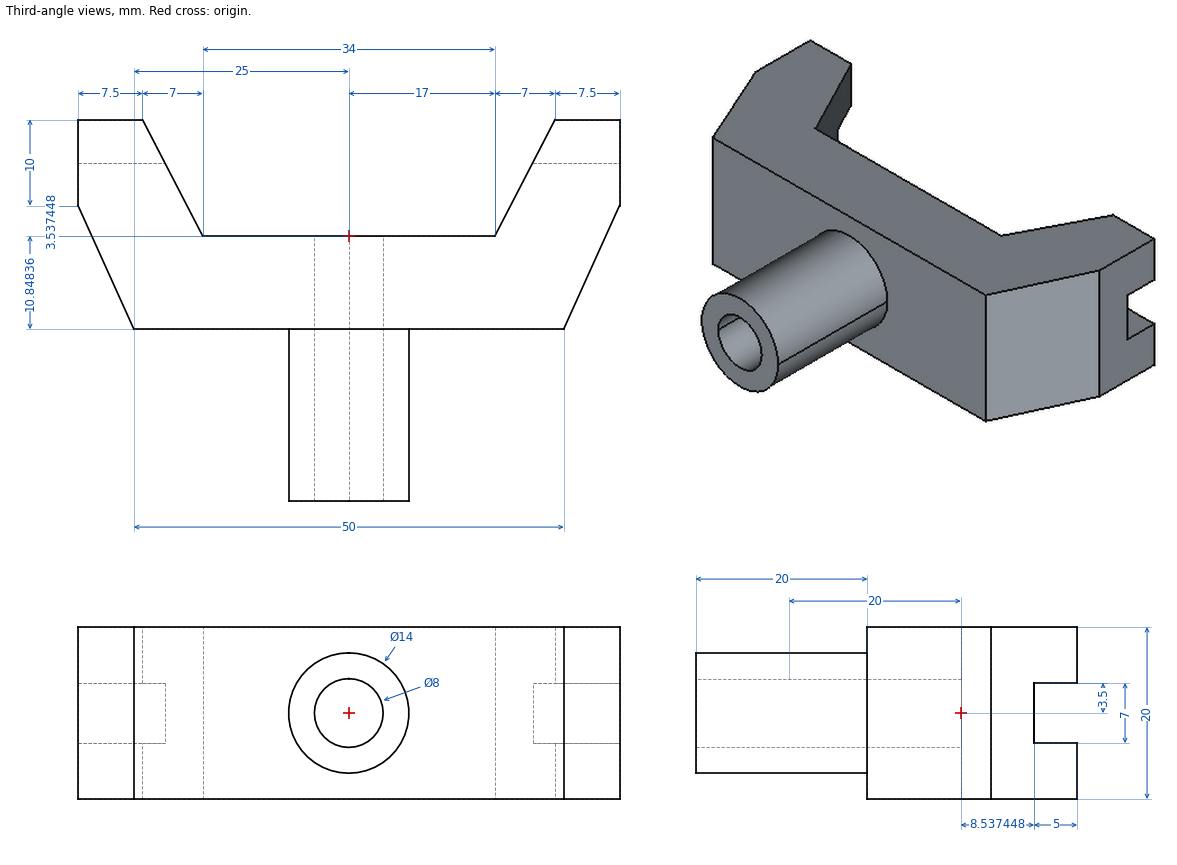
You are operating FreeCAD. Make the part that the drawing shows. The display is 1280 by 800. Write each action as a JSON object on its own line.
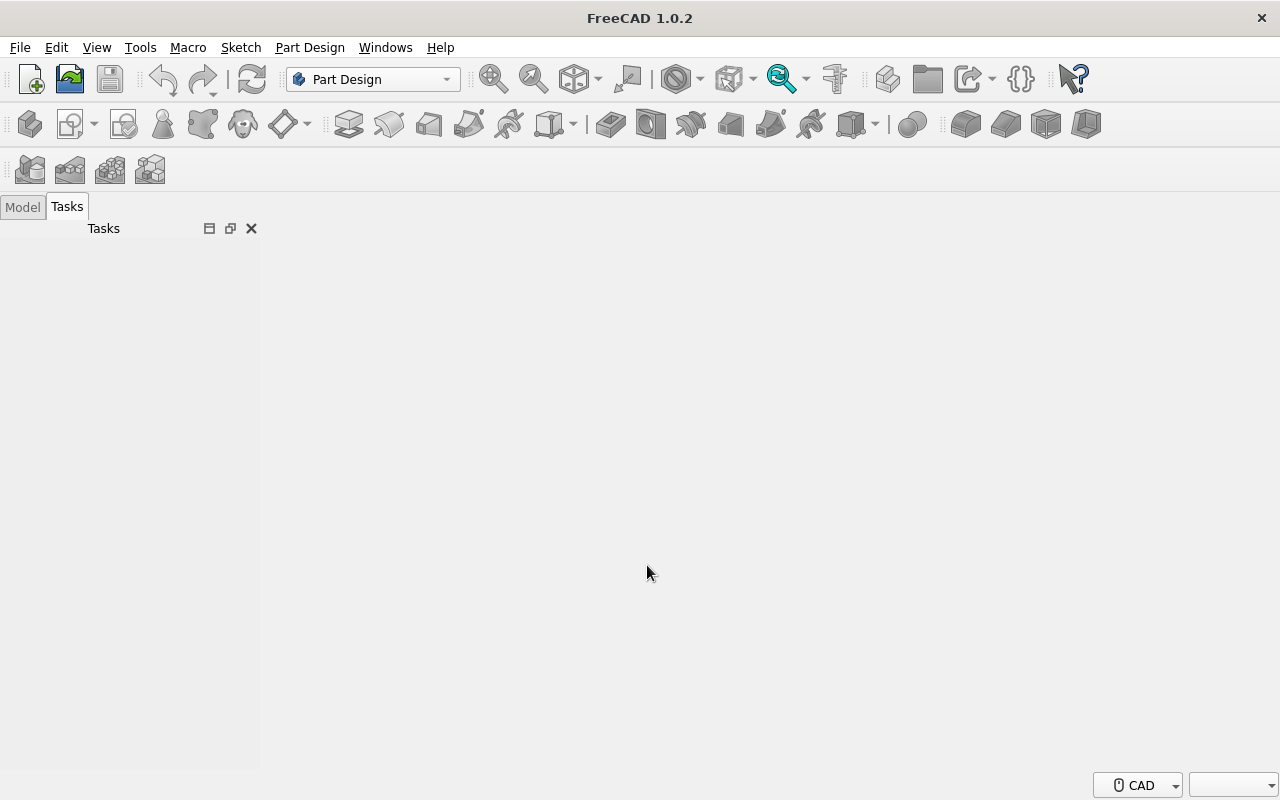
{"action": "left_click", "coordinate": [30, 80]}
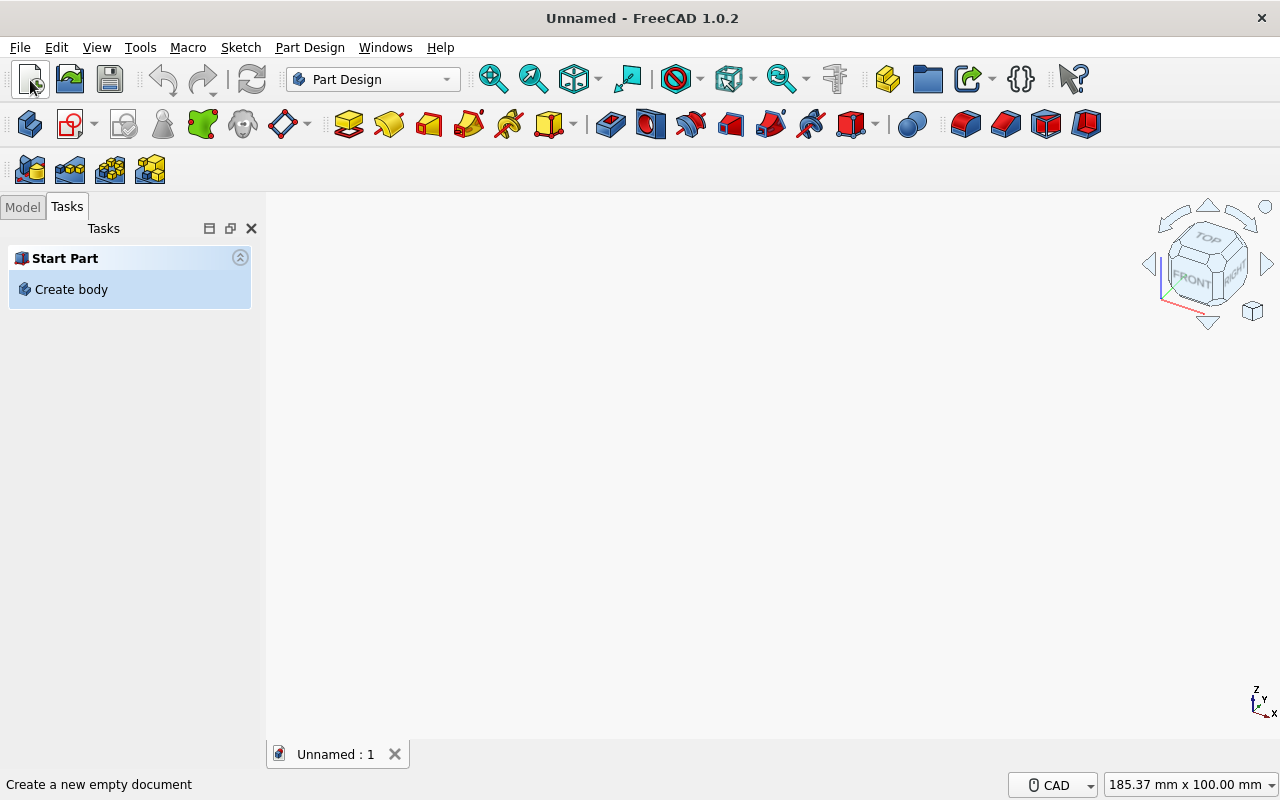
{"action": "left_click", "coordinate": [70, 124]}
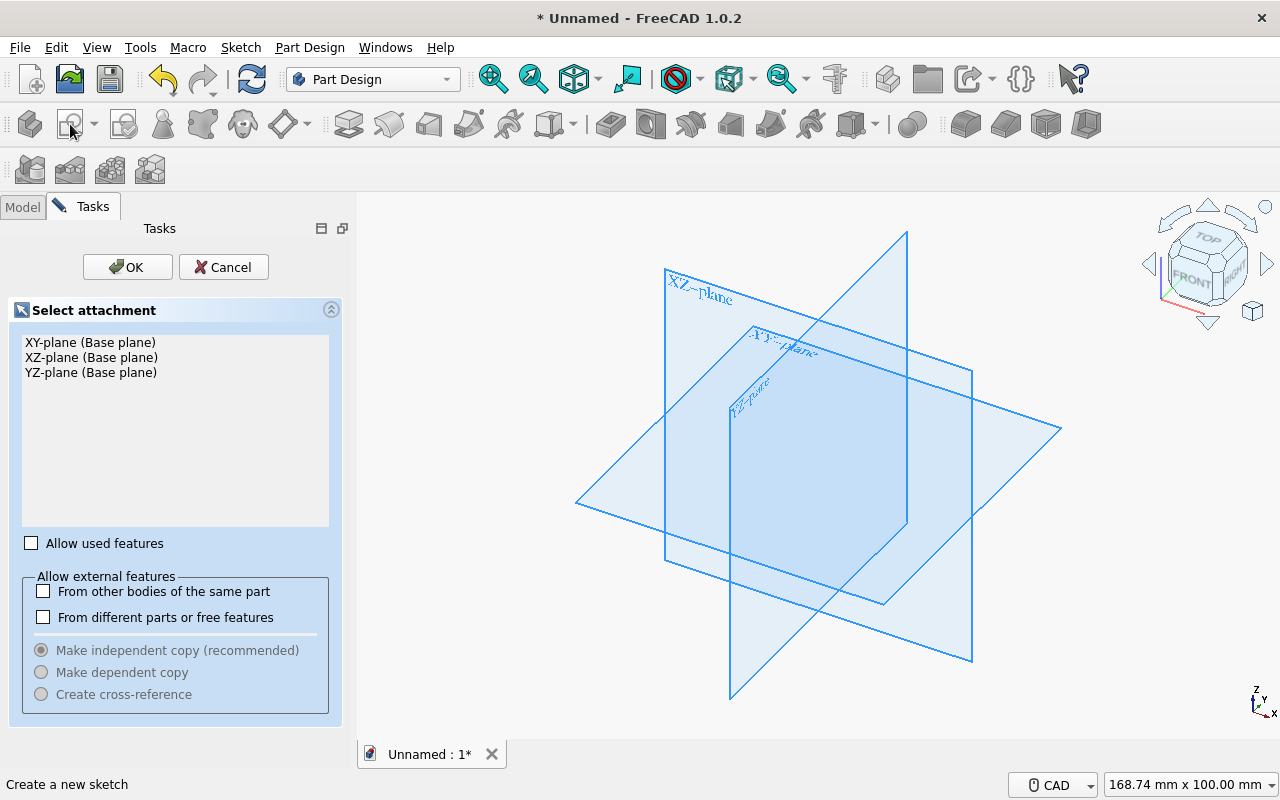
{"action": "left_click", "coordinate": [82, 342]}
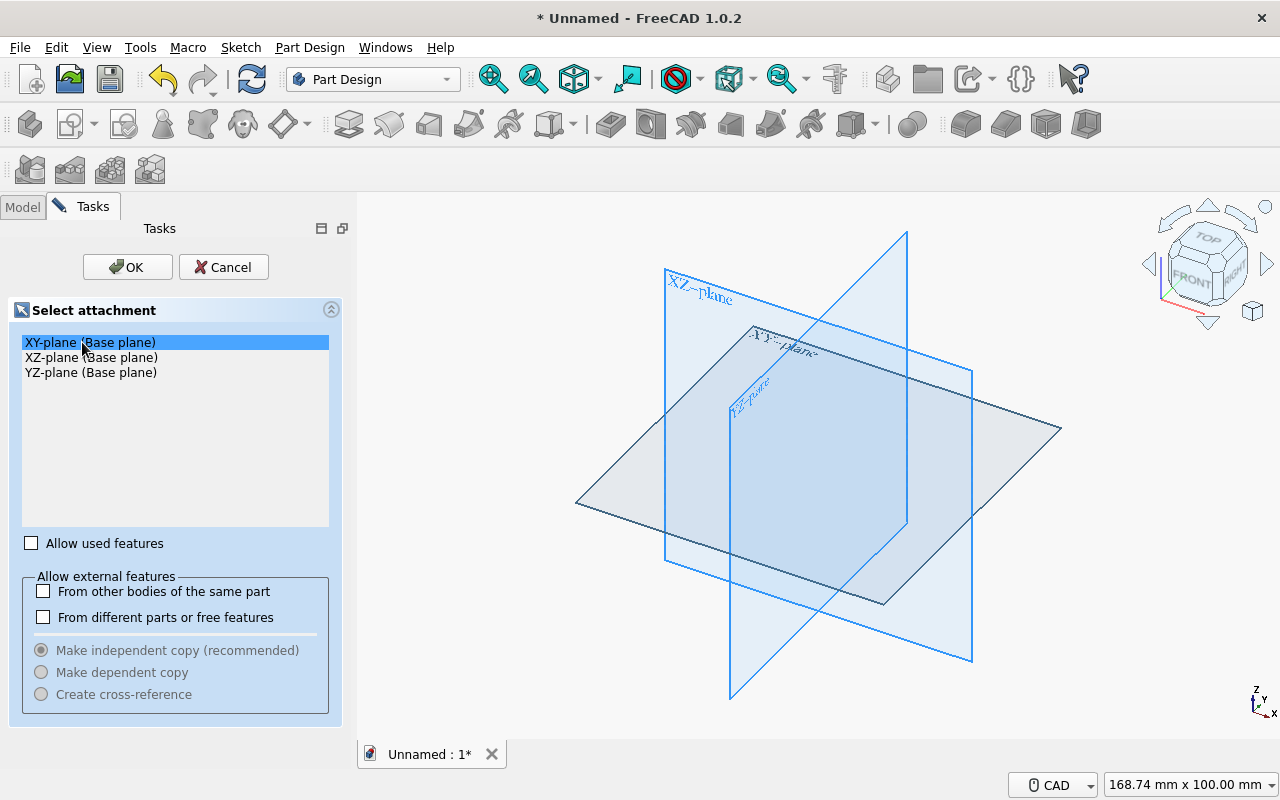
{"action": "left_click", "coordinate": [128, 267]}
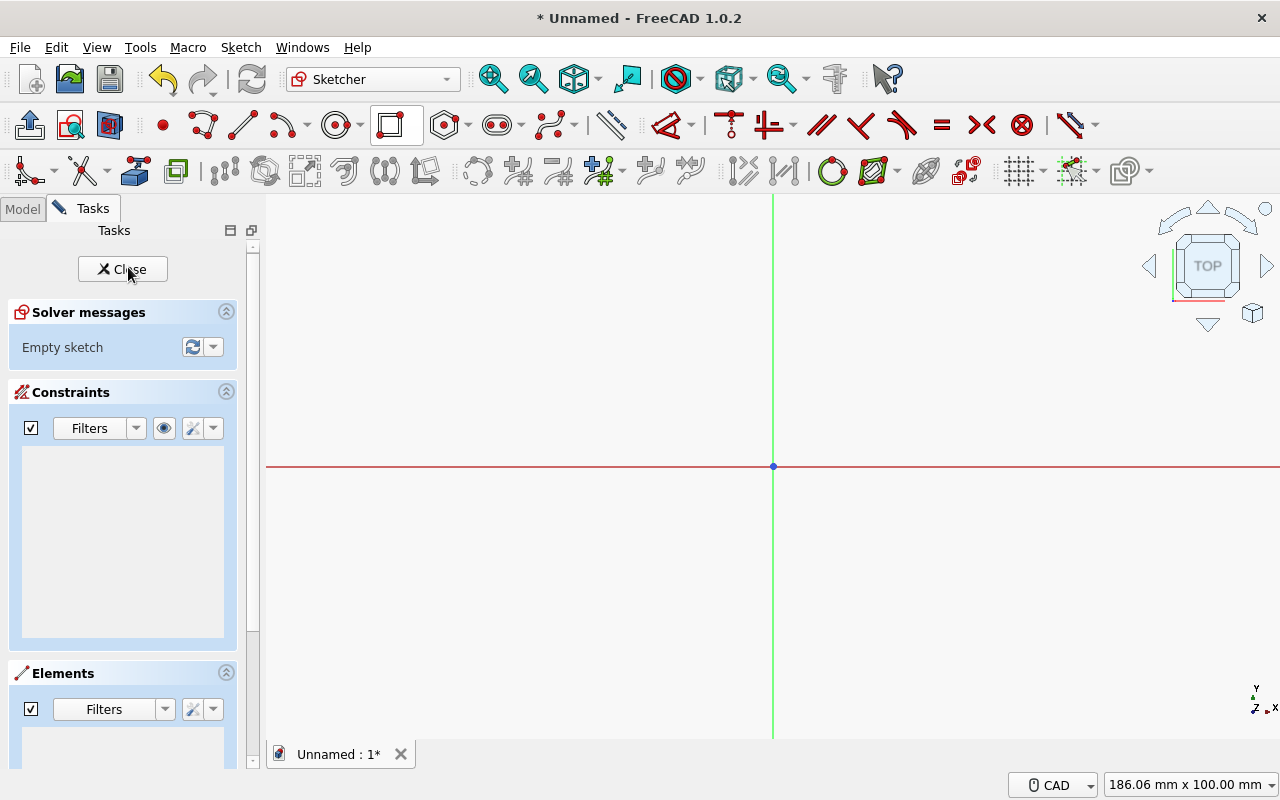
{"action": "scroll", "coordinate": [856, 450], "scroll_direction": "up", "scroll_amount": 3}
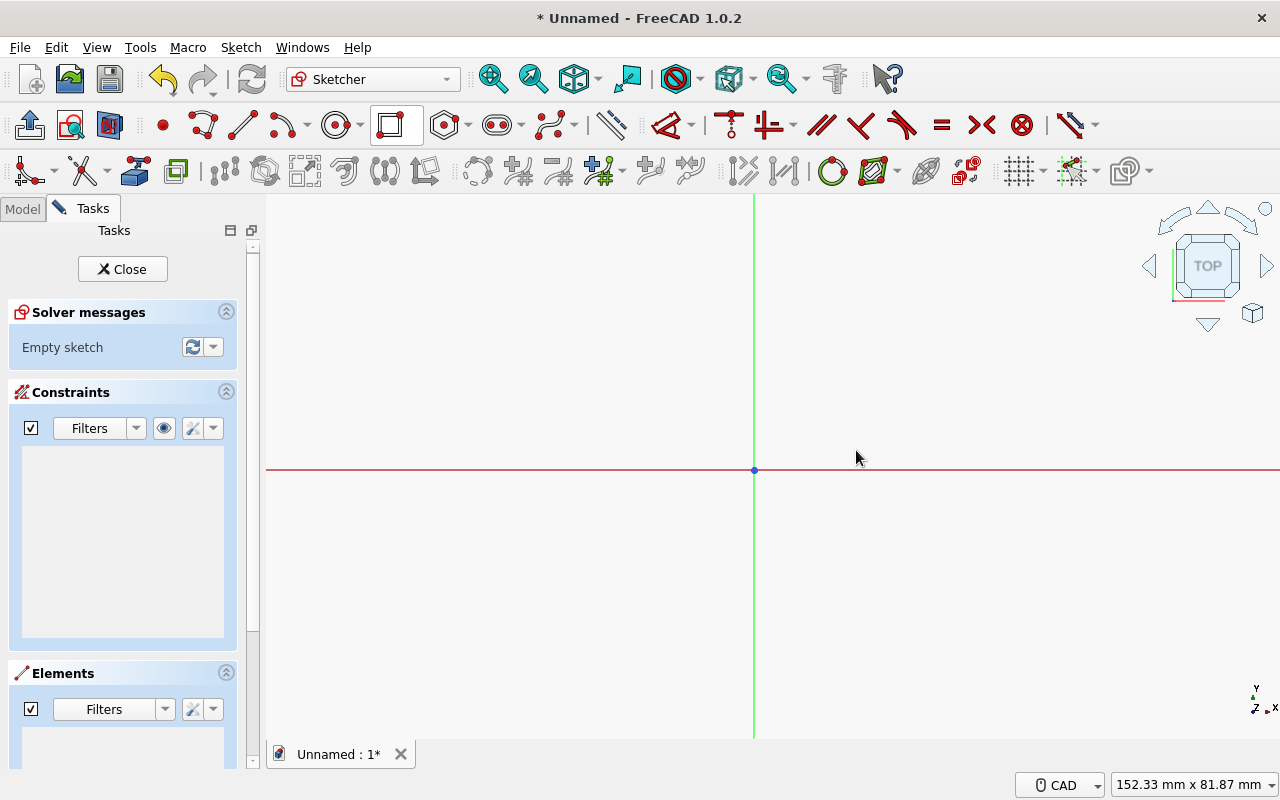
{"action": "left_click", "coordinate": [204, 126]}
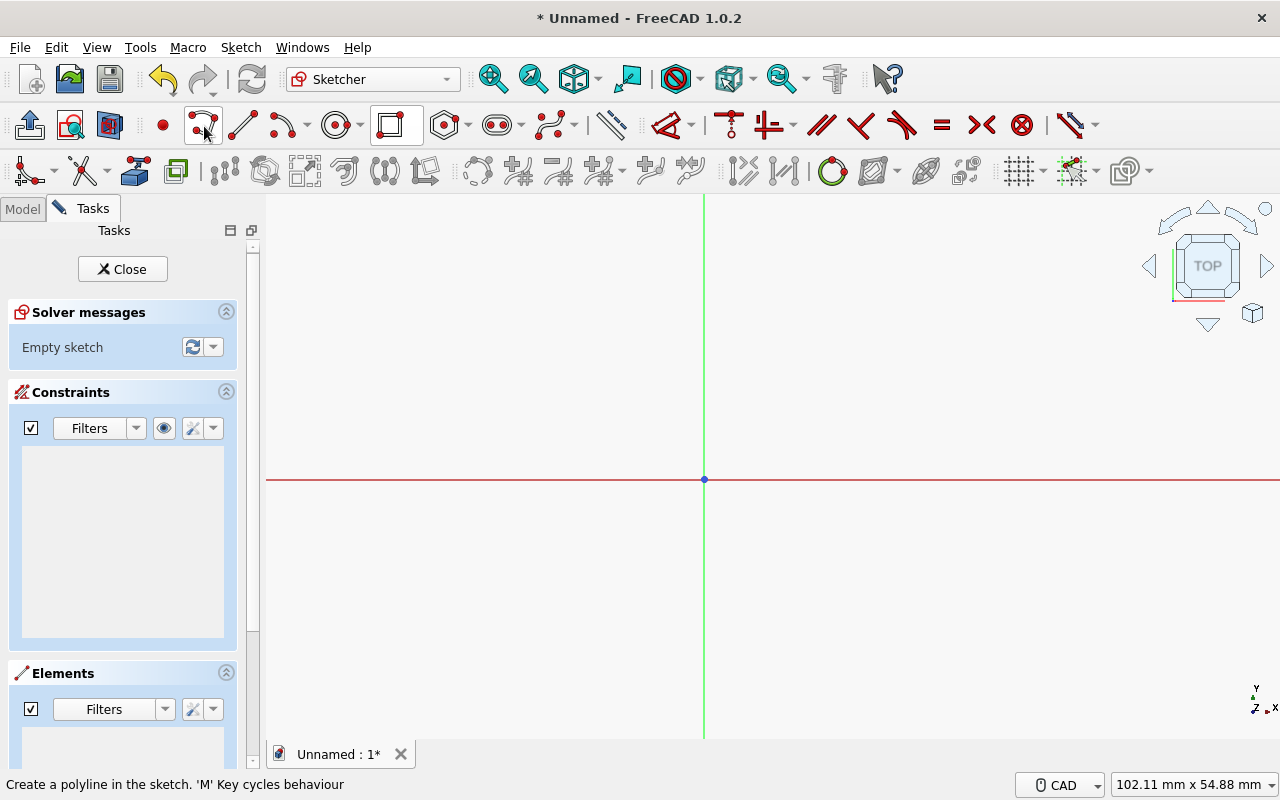
{"action": "left_click", "coordinate": [873, 480]}
{"action": "left_click", "coordinate": [535, 471]}
{"action": "left_click", "coordinate": [466, 345]}
{"action": "left_click", "coordinate": [391, 345]}
{"action": "left_click", "coordinate": [391, 445]}
{"action": "left_click", "coordinate": [456, 587]}
{"action": "left_click", "coordinate": [953, 587]}
{"action": "left_click", "coordinate": [1017, 445]}
{"action": "left_click", "coordinate": [1017, 345]}
{"action": "left_click", "coordinate": [943, 345]}
{"action": "left_click", "coordinate": [873, 480]}
{"action": "key", "text": "Escape"}
{"action": "key", "text": "Escape"}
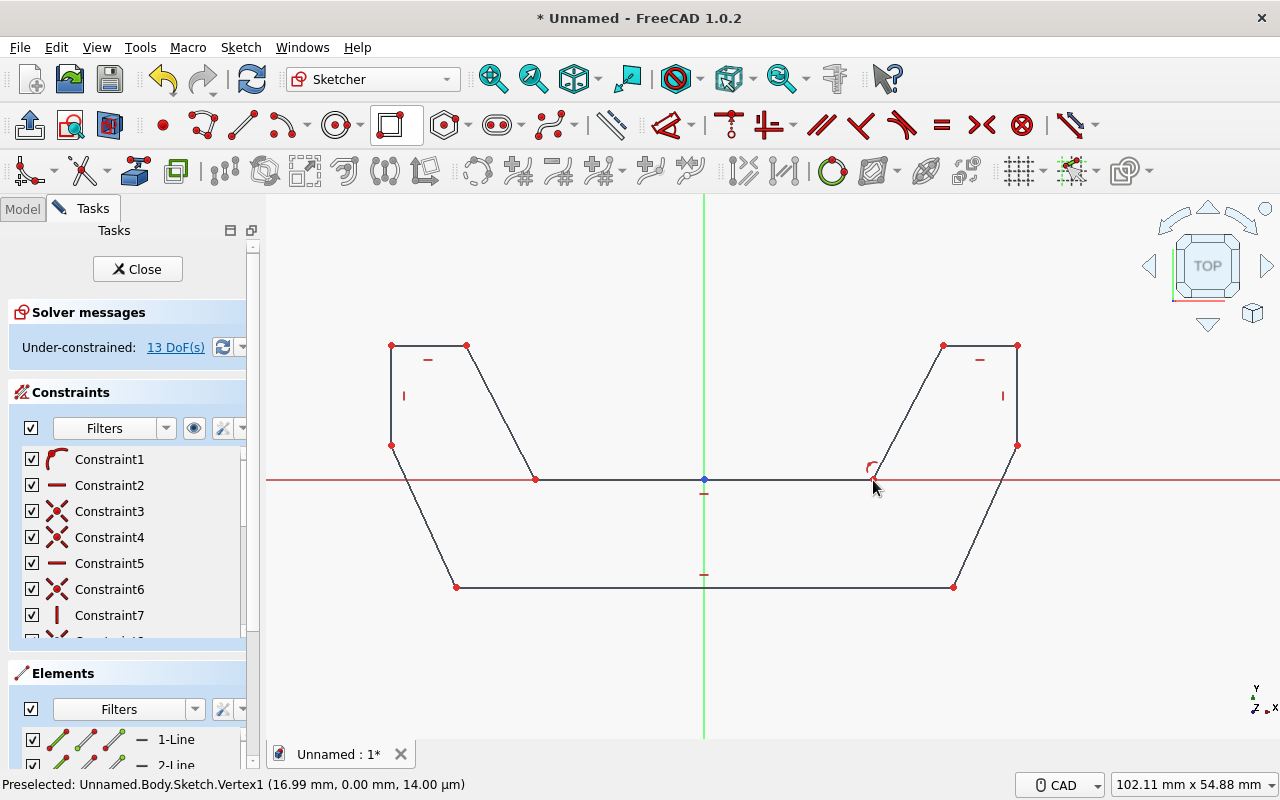
{"action": "left_click", "coordinate": [666, 126]}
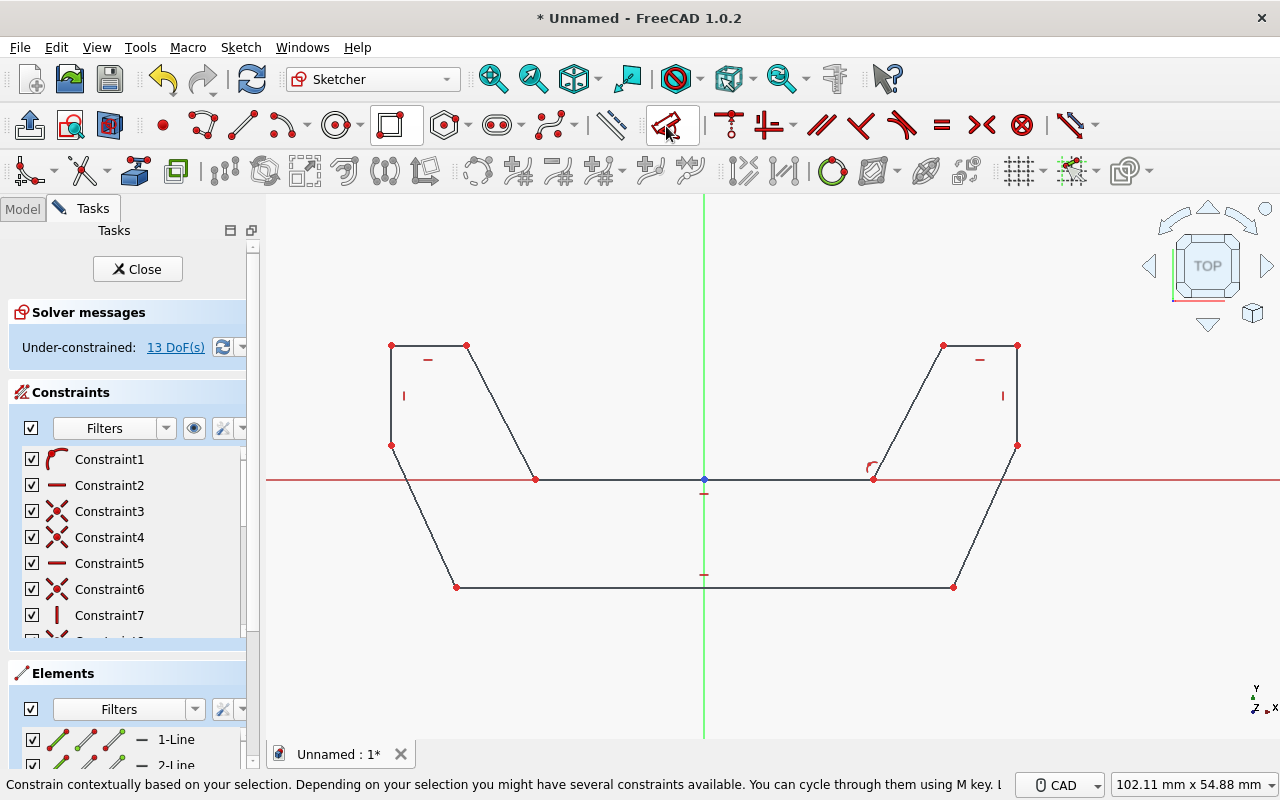
{"action": "left_click", "coordinate": [772, 480]}
{"action": "left_click", "coordinate": [626, 514]}